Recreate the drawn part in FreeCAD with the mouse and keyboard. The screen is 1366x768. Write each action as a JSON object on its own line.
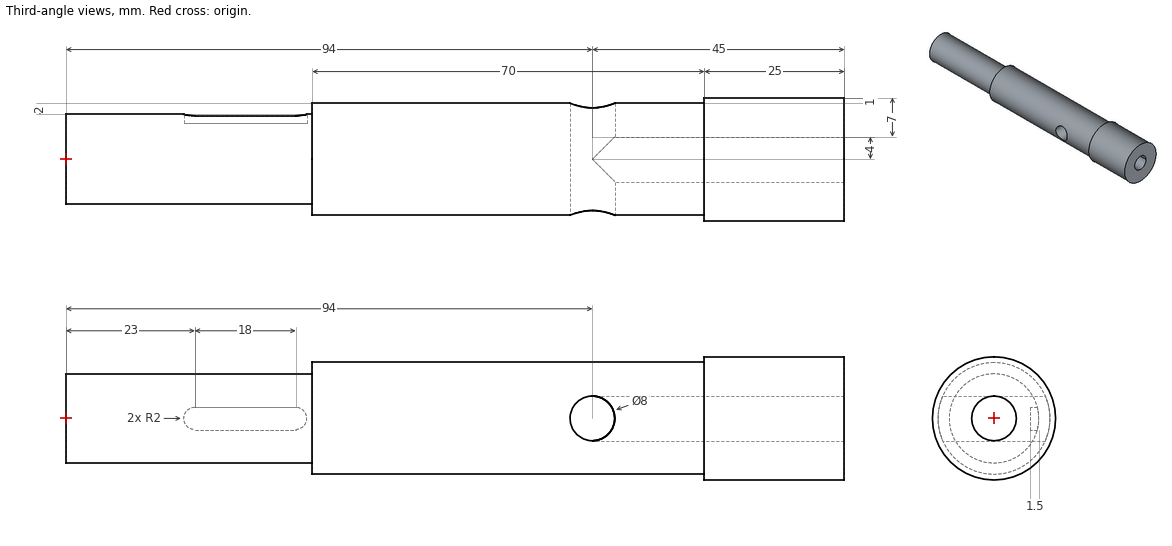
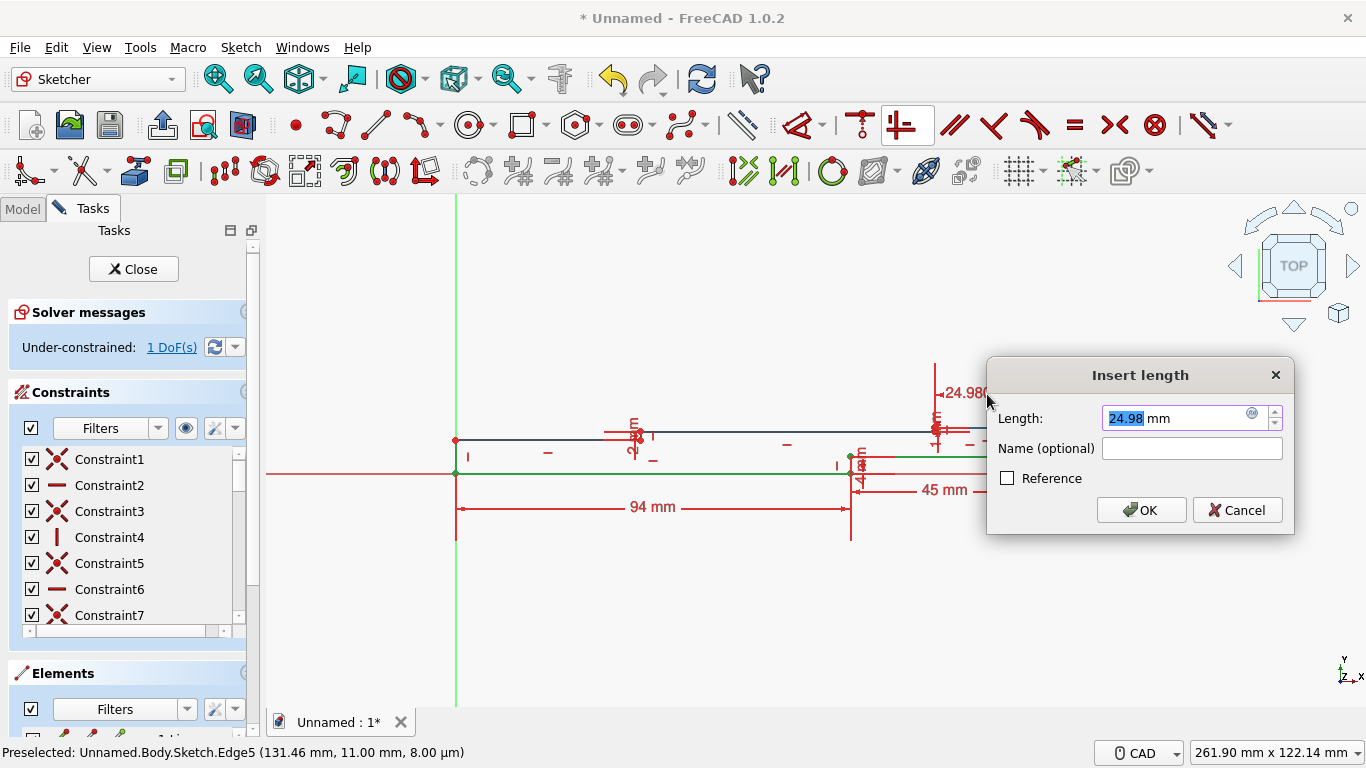
{"action": "type", "text": "25"}
{"action": "key", "text": "Return"}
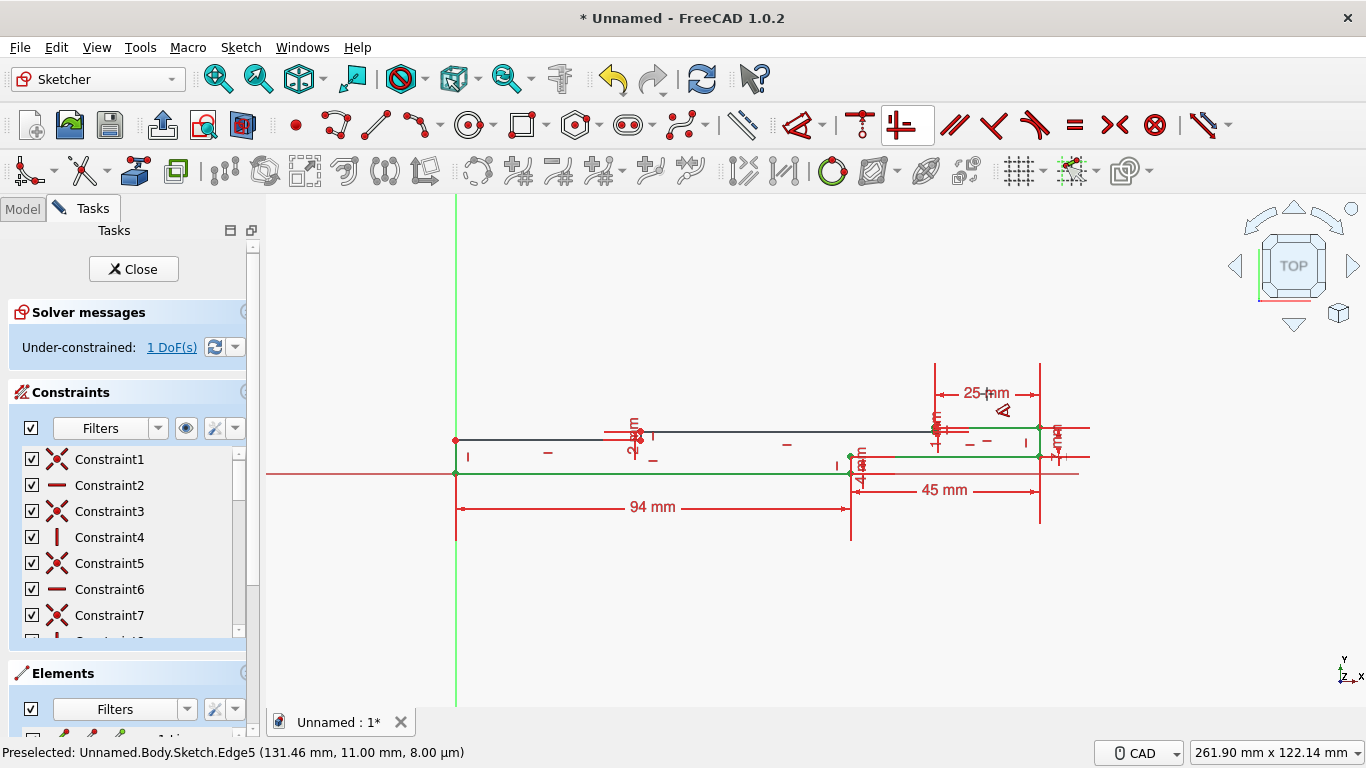
{"action": "left_click", "coordinate": [847, 432]}
{"action": "left_click", "coordinate": [788, 398]}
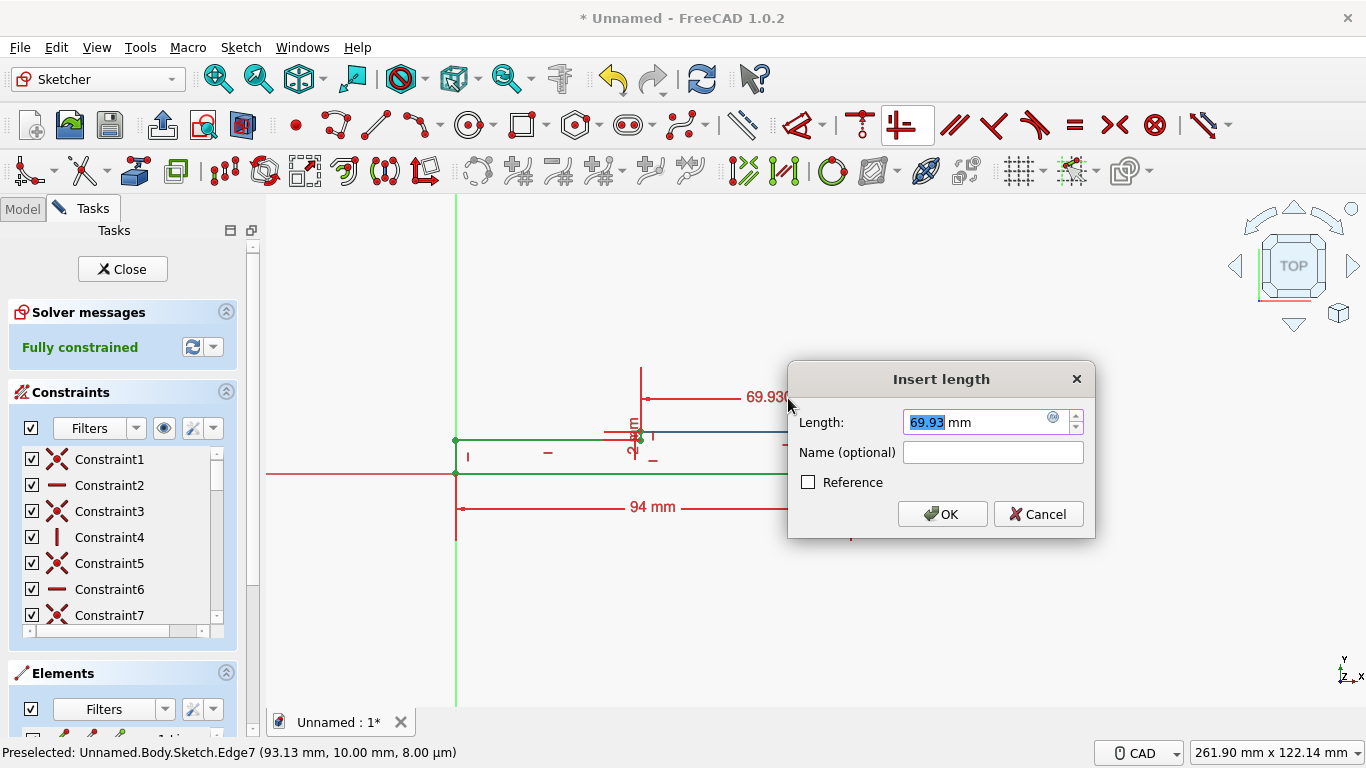
{"action": "type", "text": "70"}
{"action": "key", "text": "Return"}
{"action": "key", "text": "Escape"}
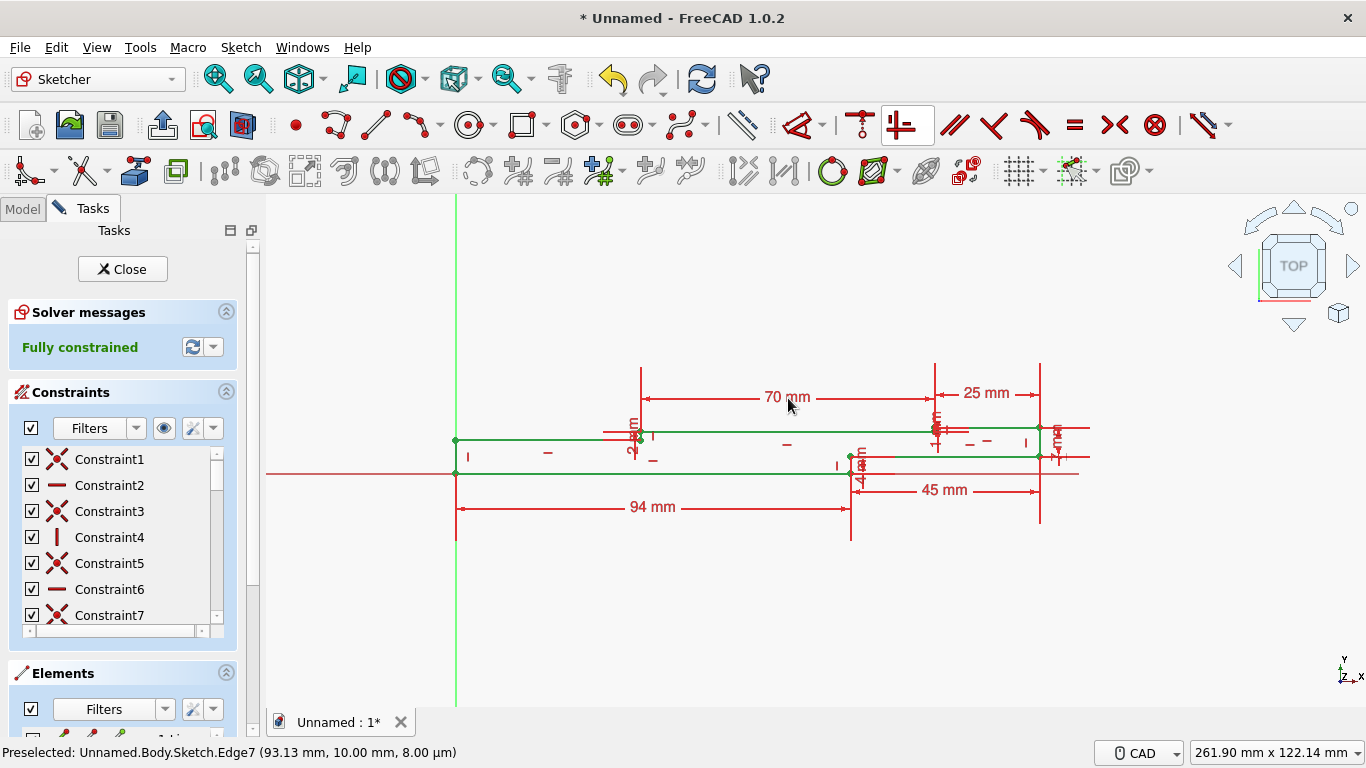
{"action": "left_click", "coordinate": [123, 269]}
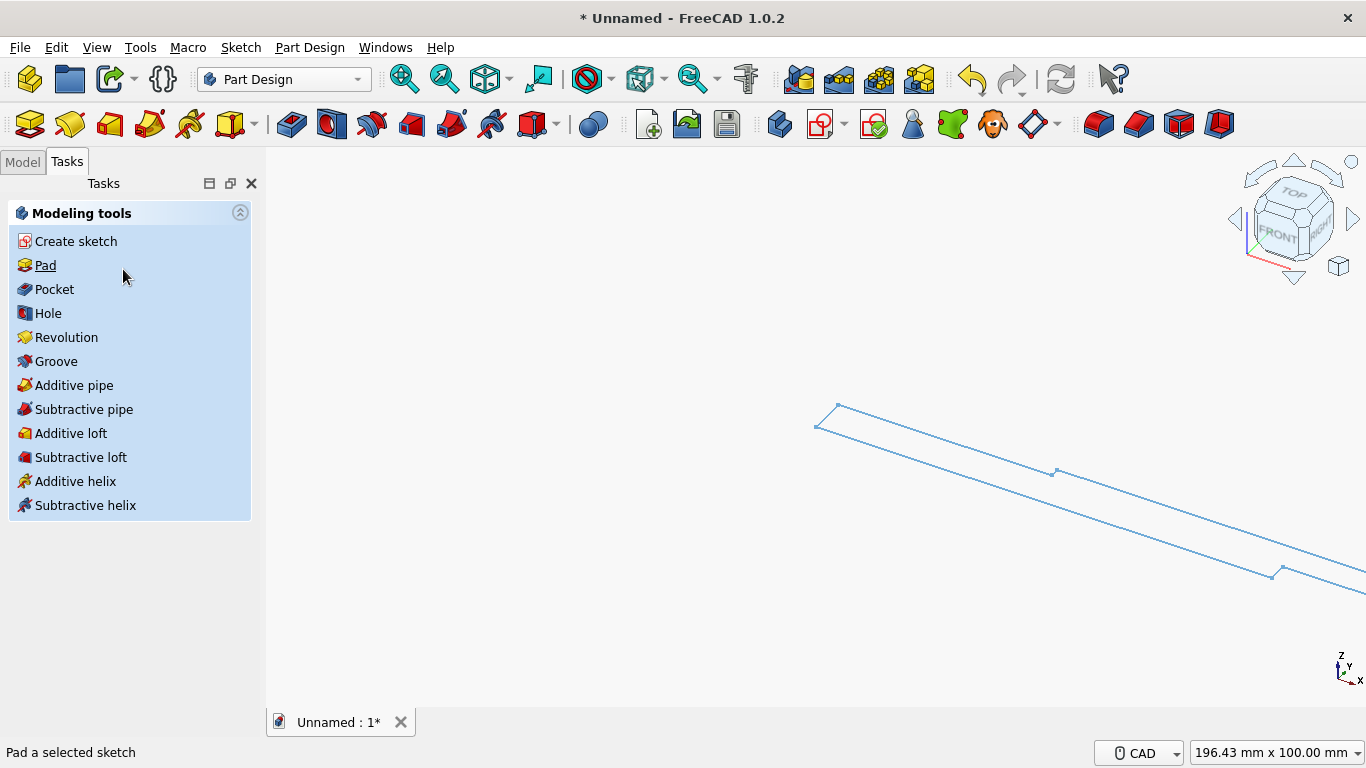
{"action": "left_click", "coordinate": [70, 124]}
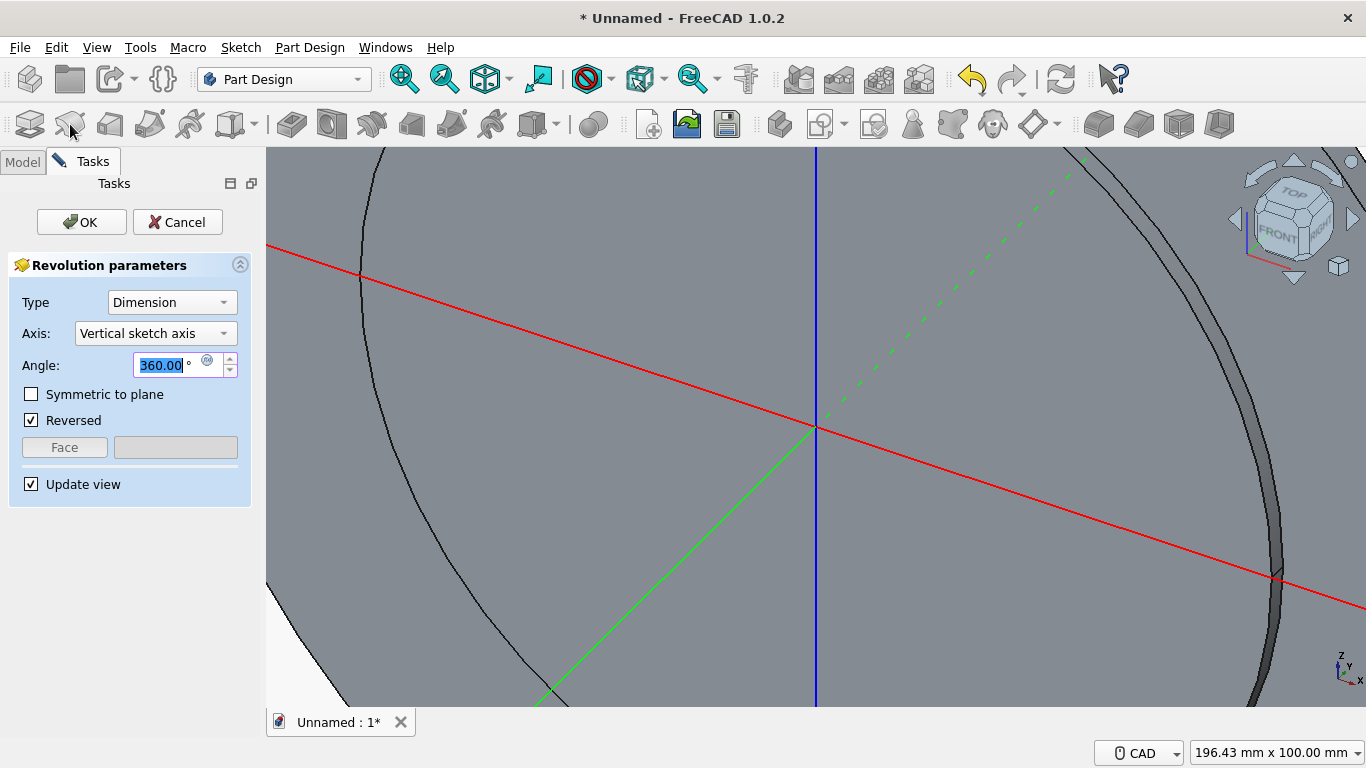
{"action": "left_click", "coordinate": [156, 334]}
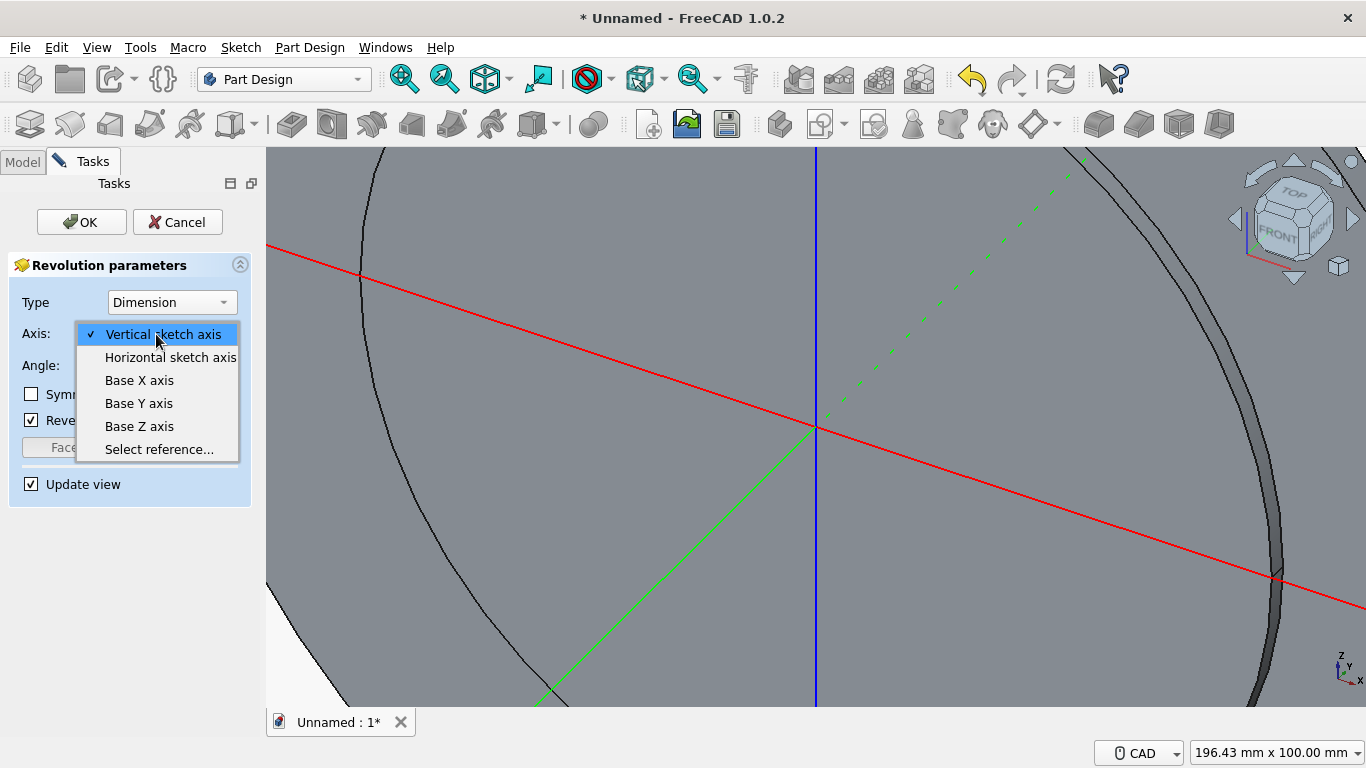
{"action": "left_click", "coordinate": [156, 358]}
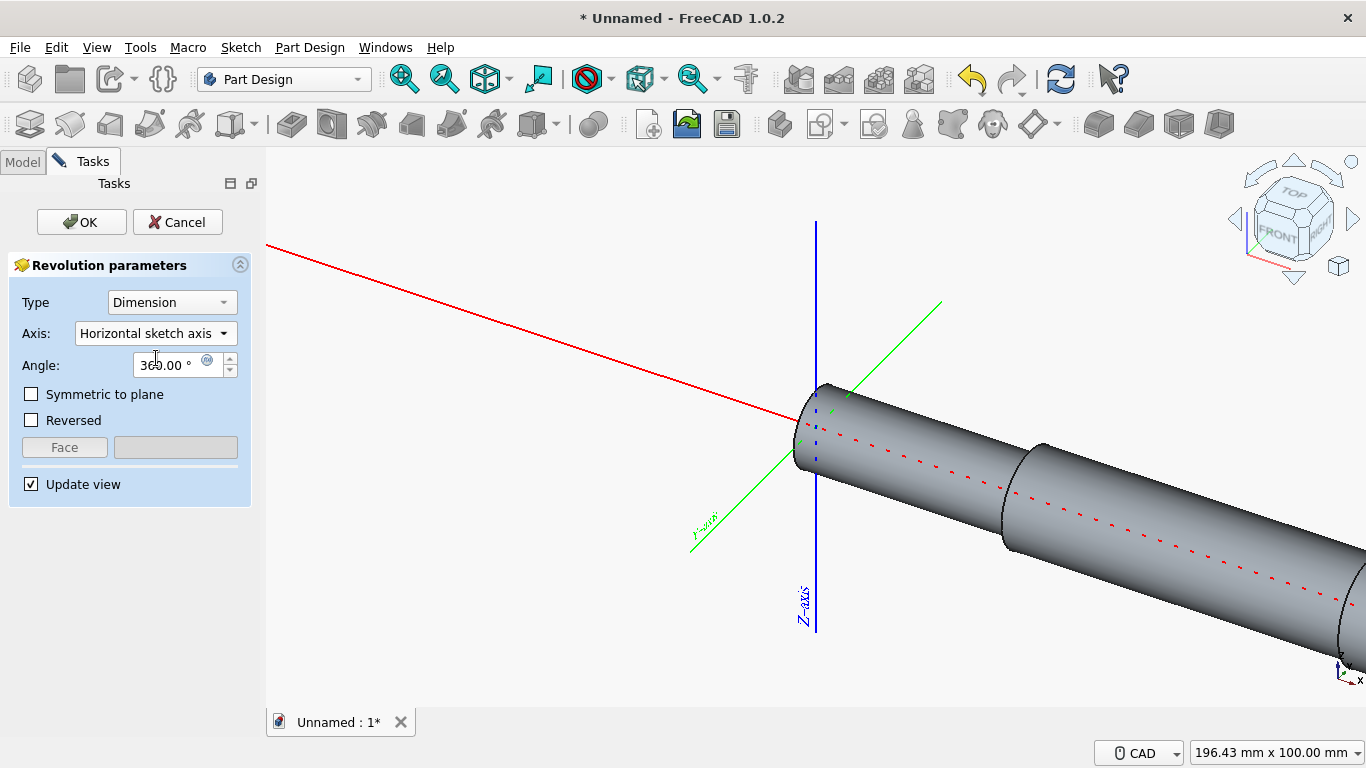
{"action": "left_click", "coordinate": [82, 222]}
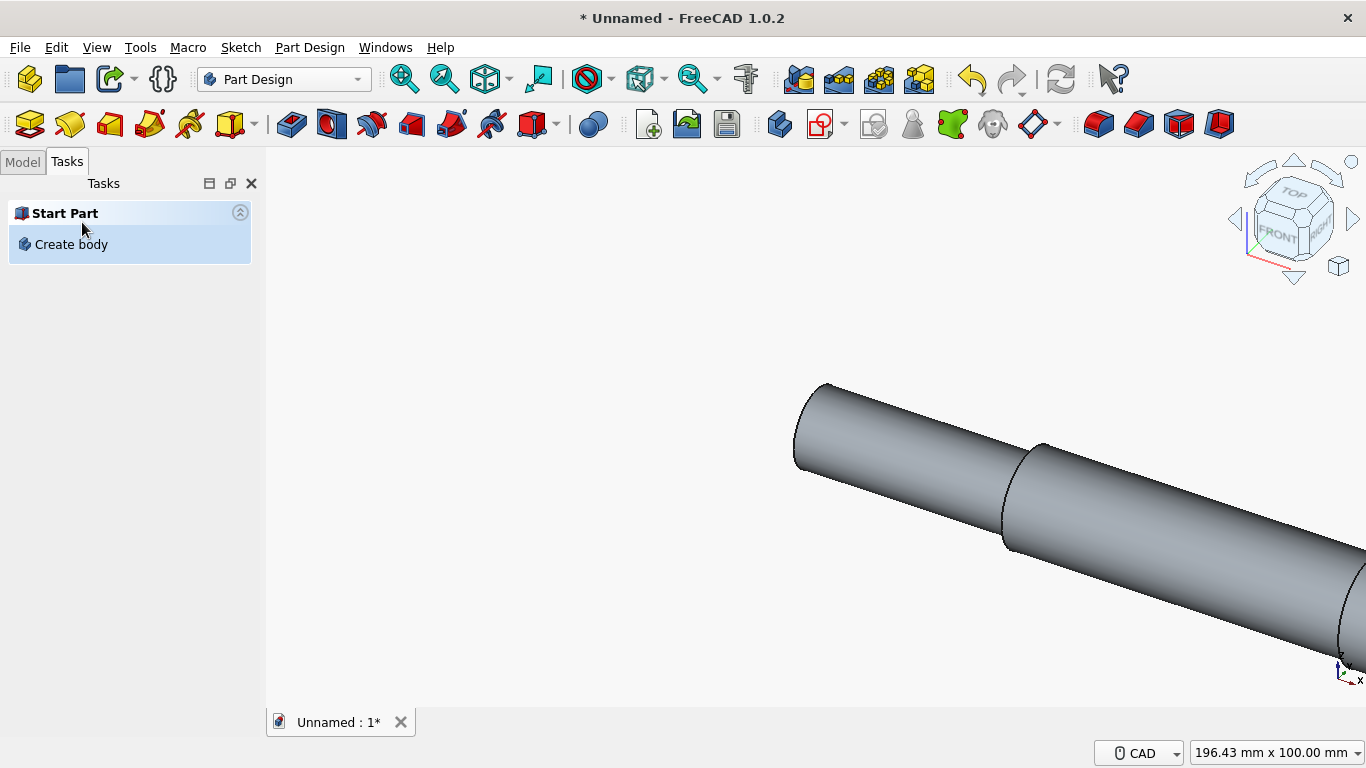
{"action": "key", "text": "v f"}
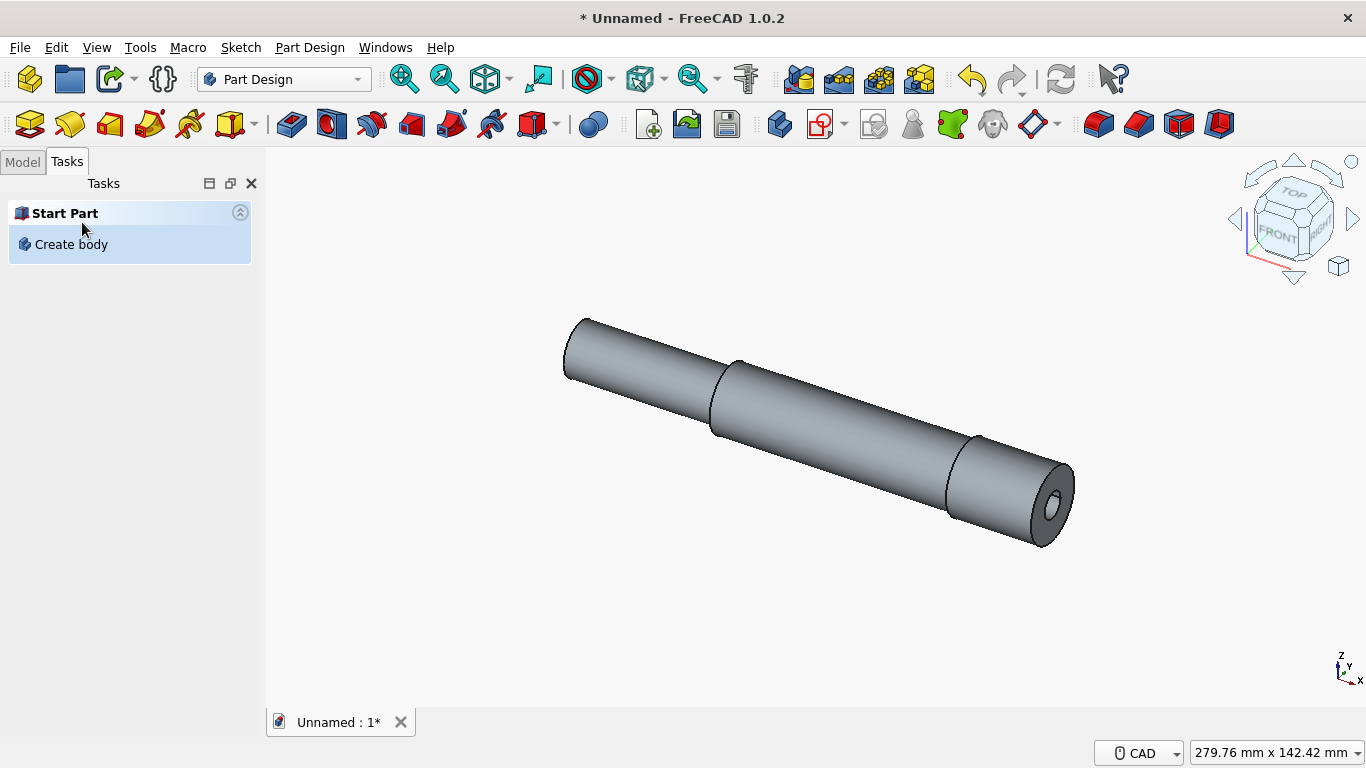
{"action": "left_click", "coordinate": [23, 161]}